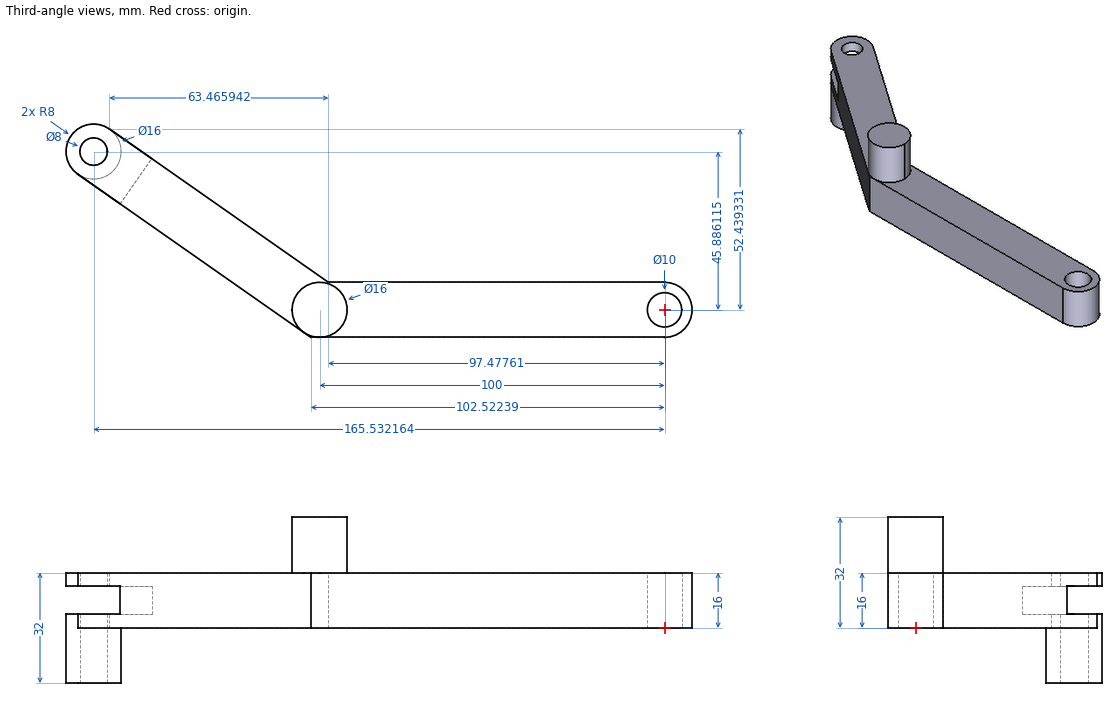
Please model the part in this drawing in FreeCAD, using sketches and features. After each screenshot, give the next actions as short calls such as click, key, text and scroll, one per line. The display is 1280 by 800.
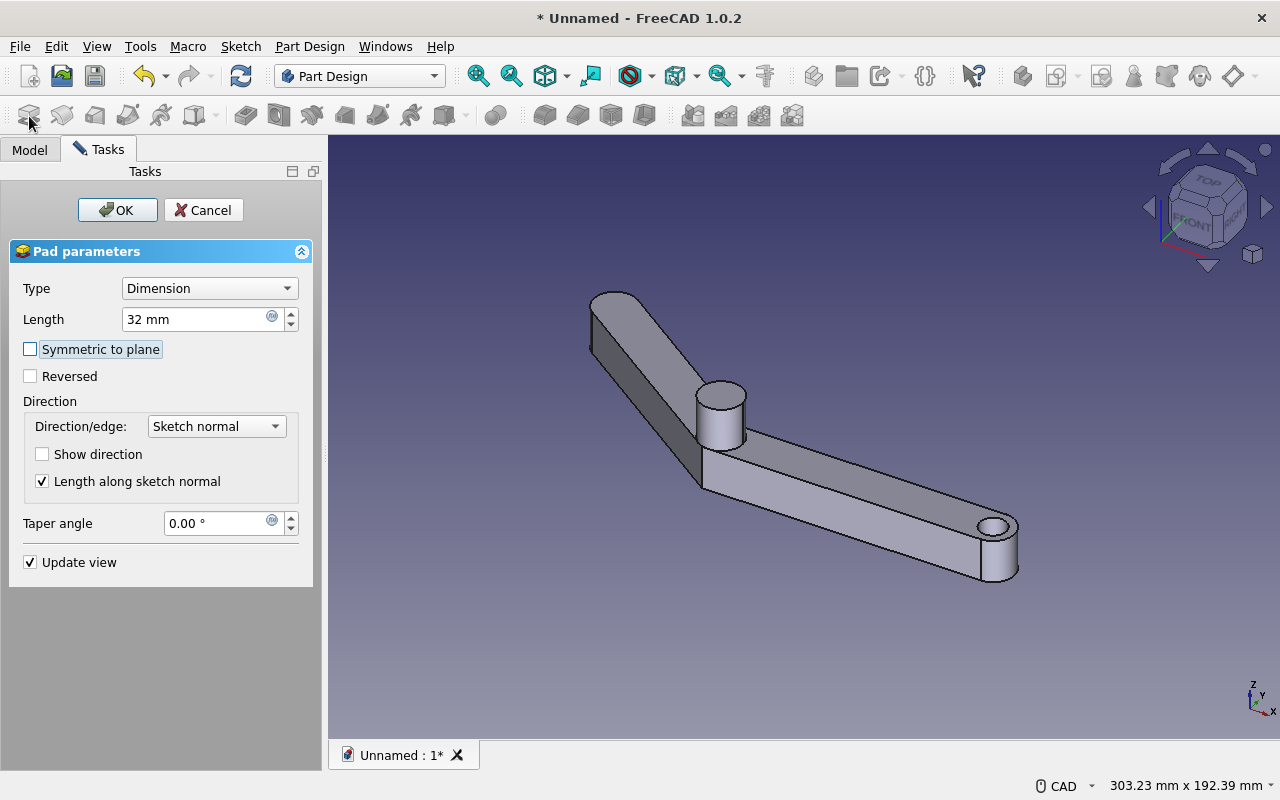
click(118, 210)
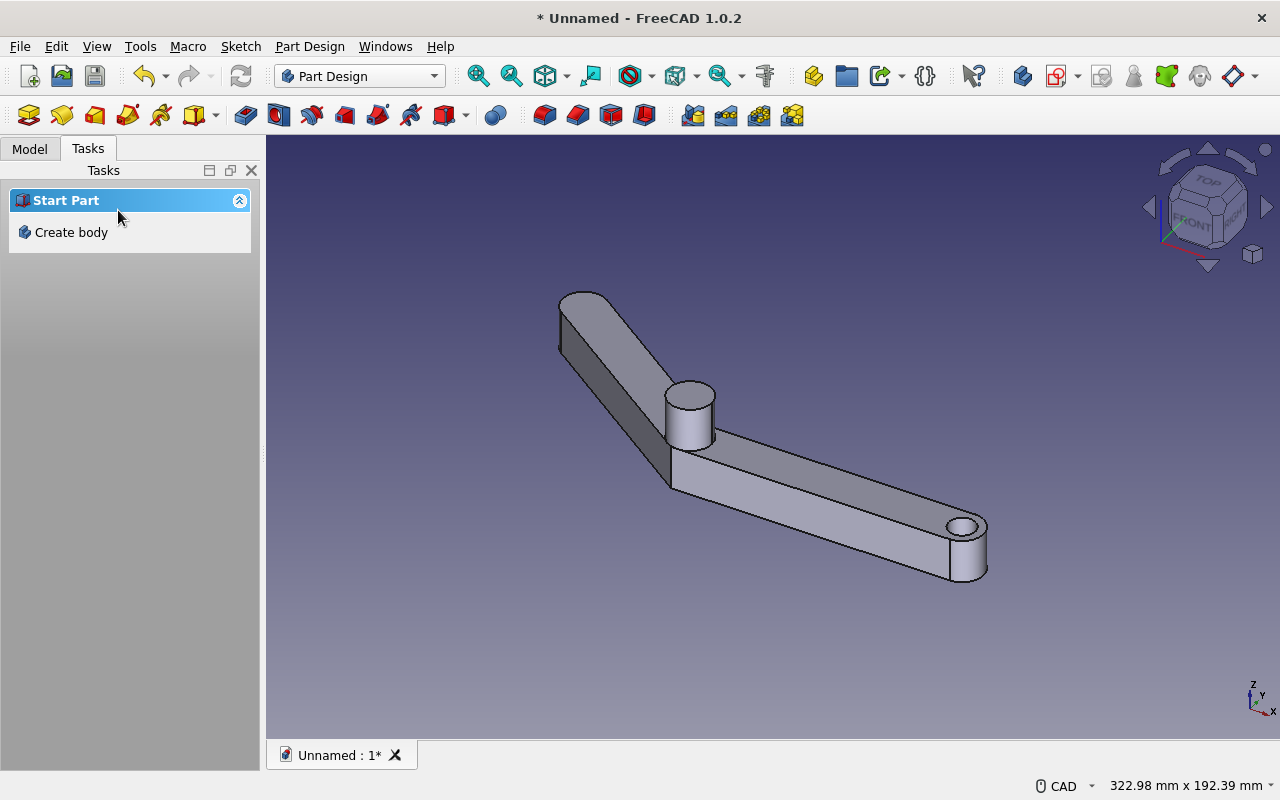
click(30, 148)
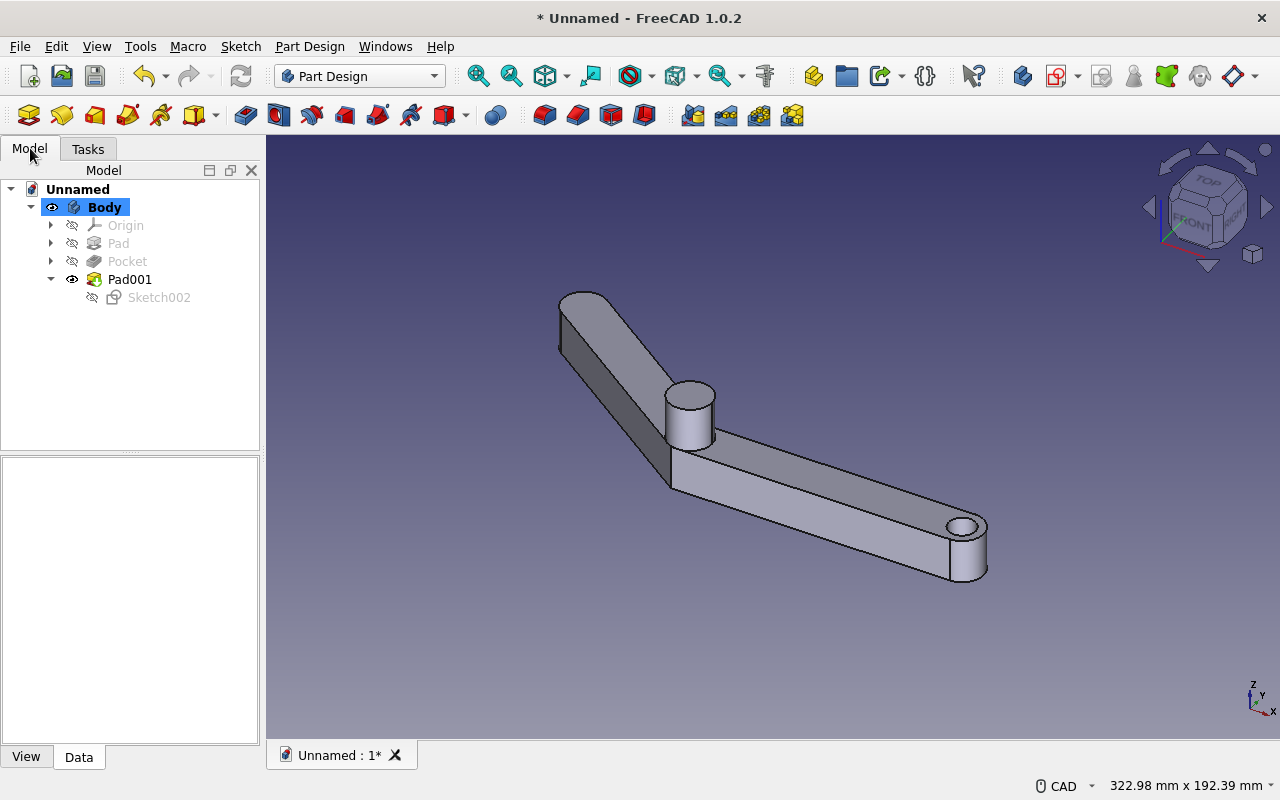
click(51, 225)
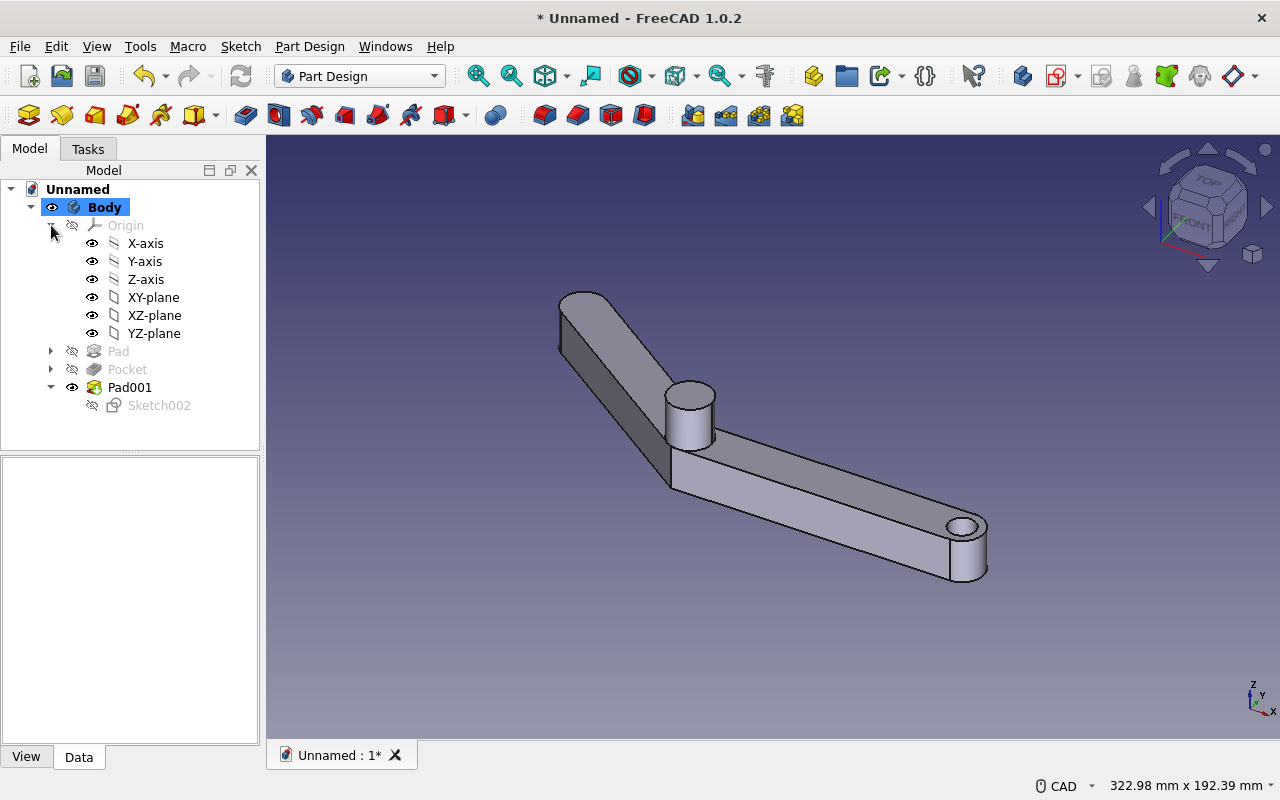
click(137, 297)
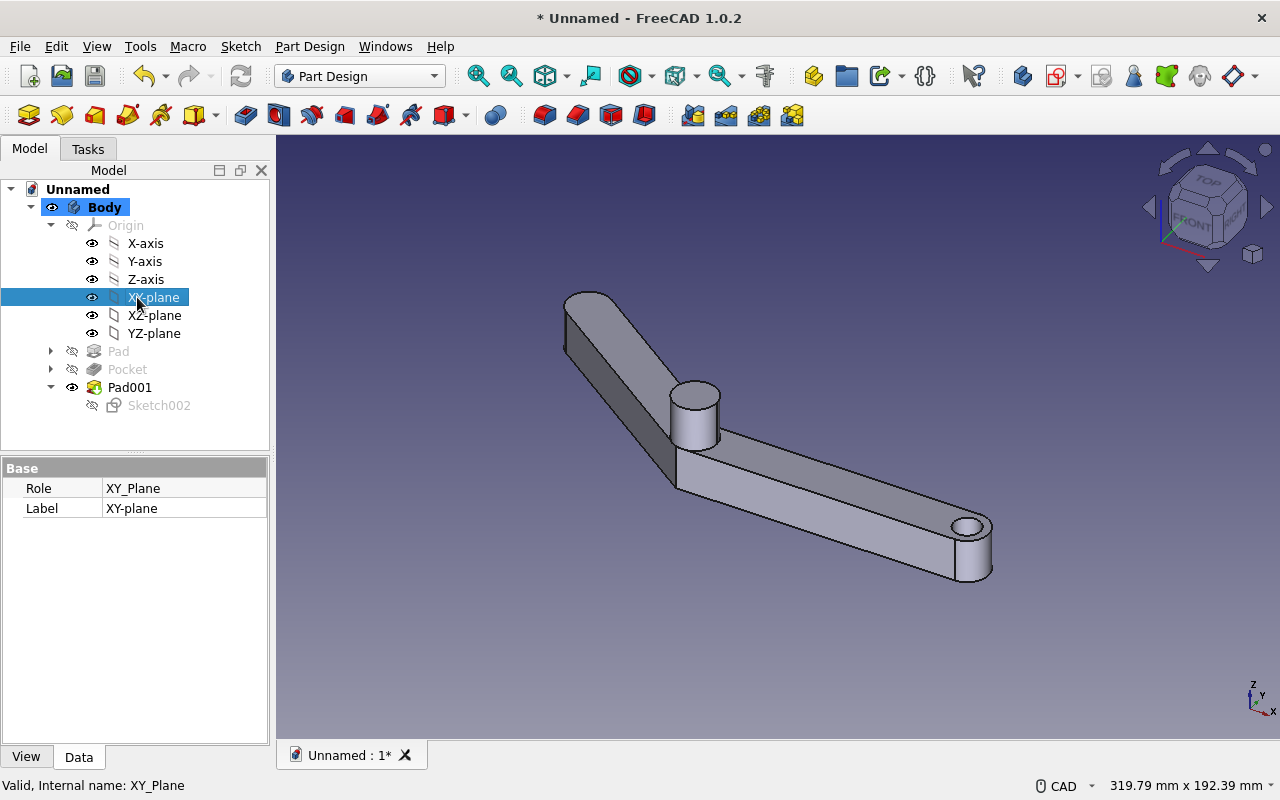
click(1232, 76)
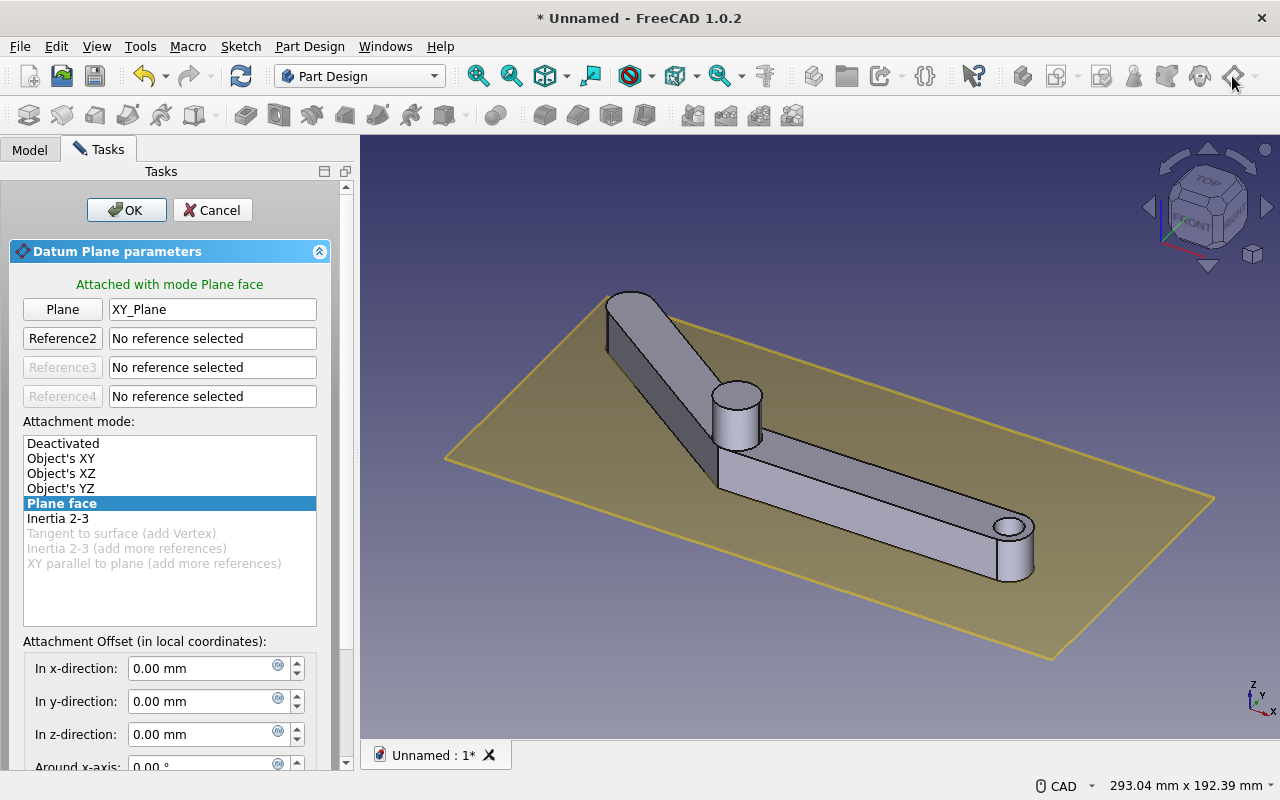
triple_click(210, 734)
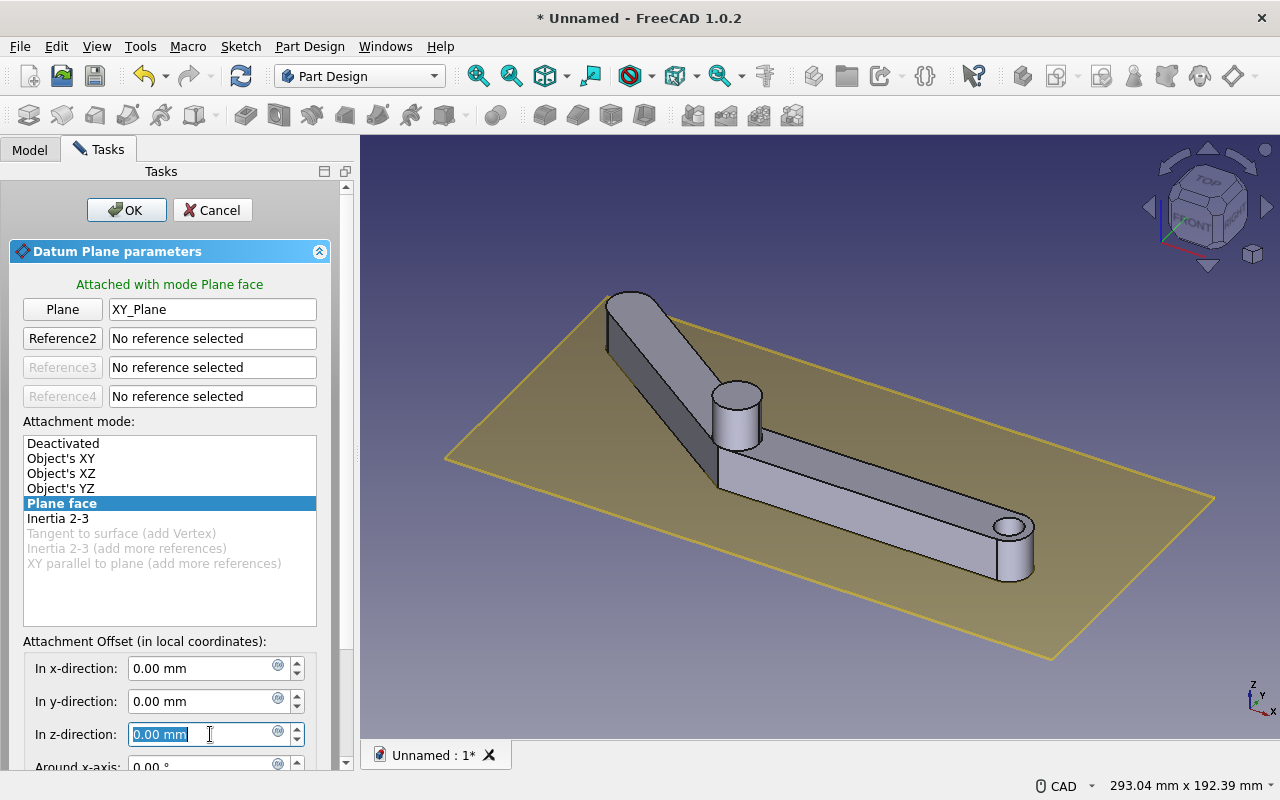
text(-16)
key(Tab)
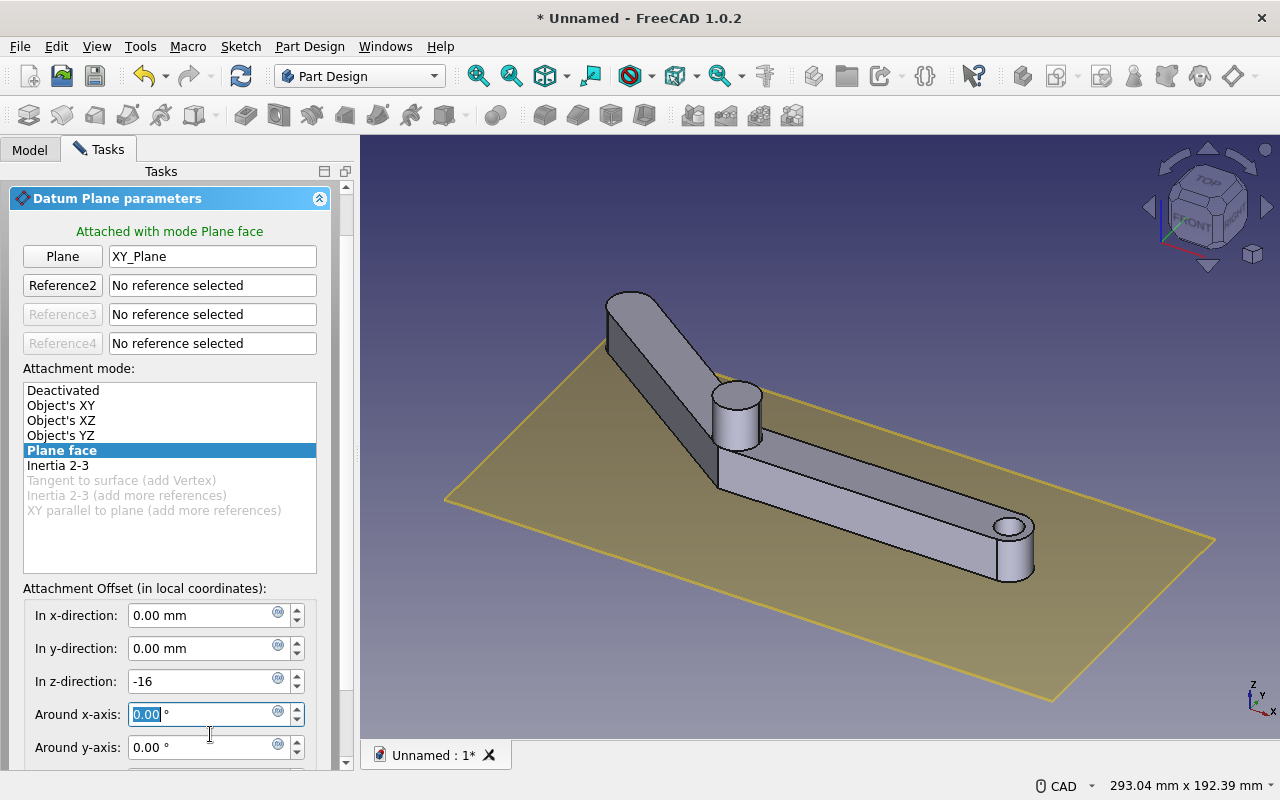
scroll(346, 476, up, 2)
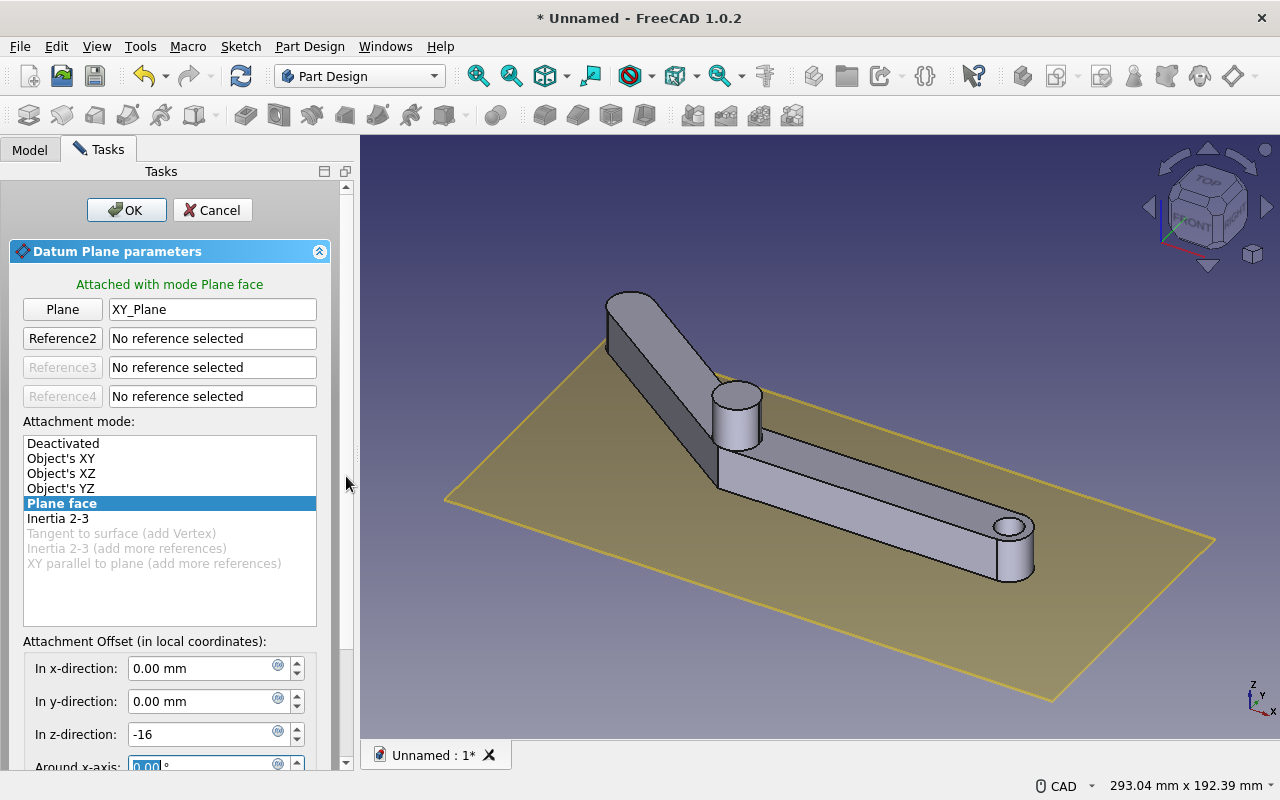
click(127, 210)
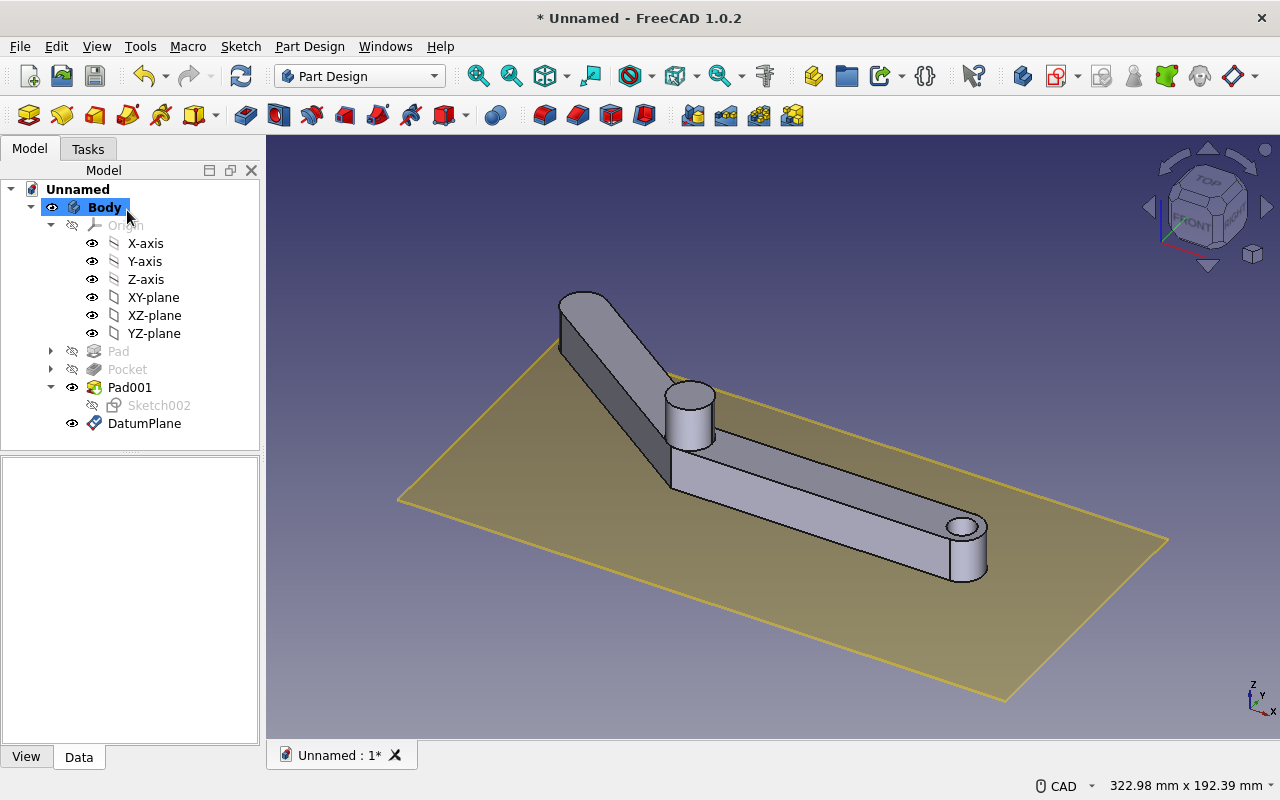
click(117, 423)